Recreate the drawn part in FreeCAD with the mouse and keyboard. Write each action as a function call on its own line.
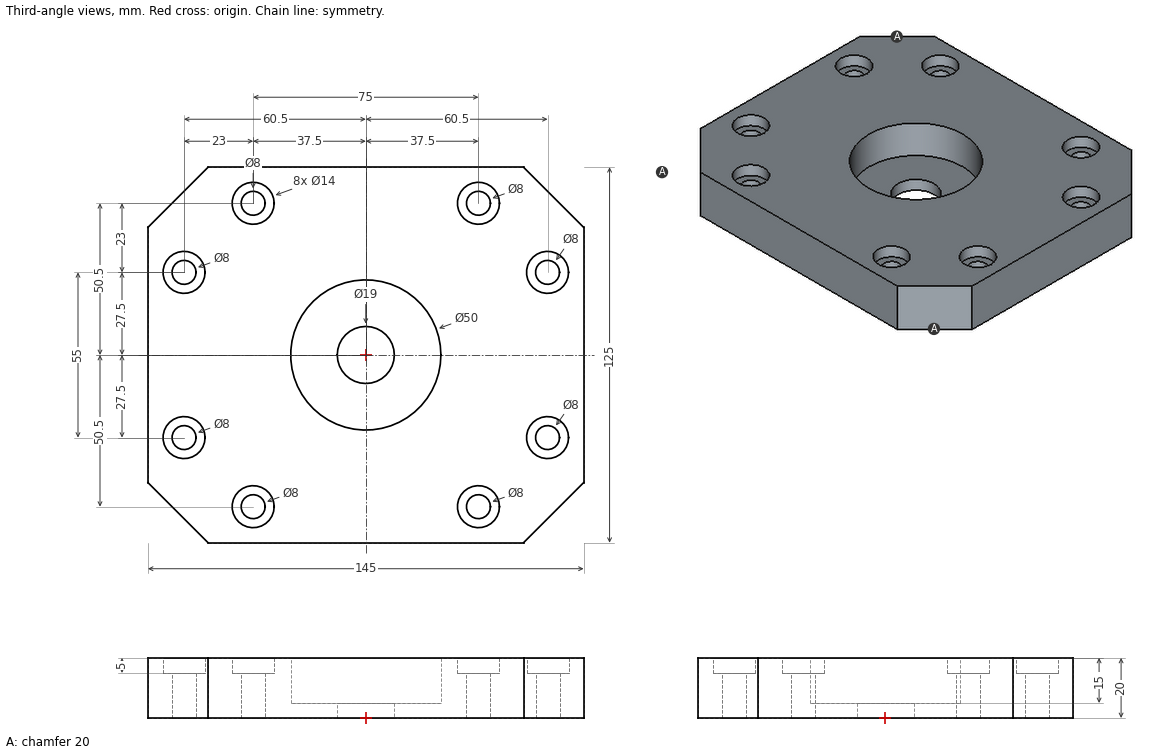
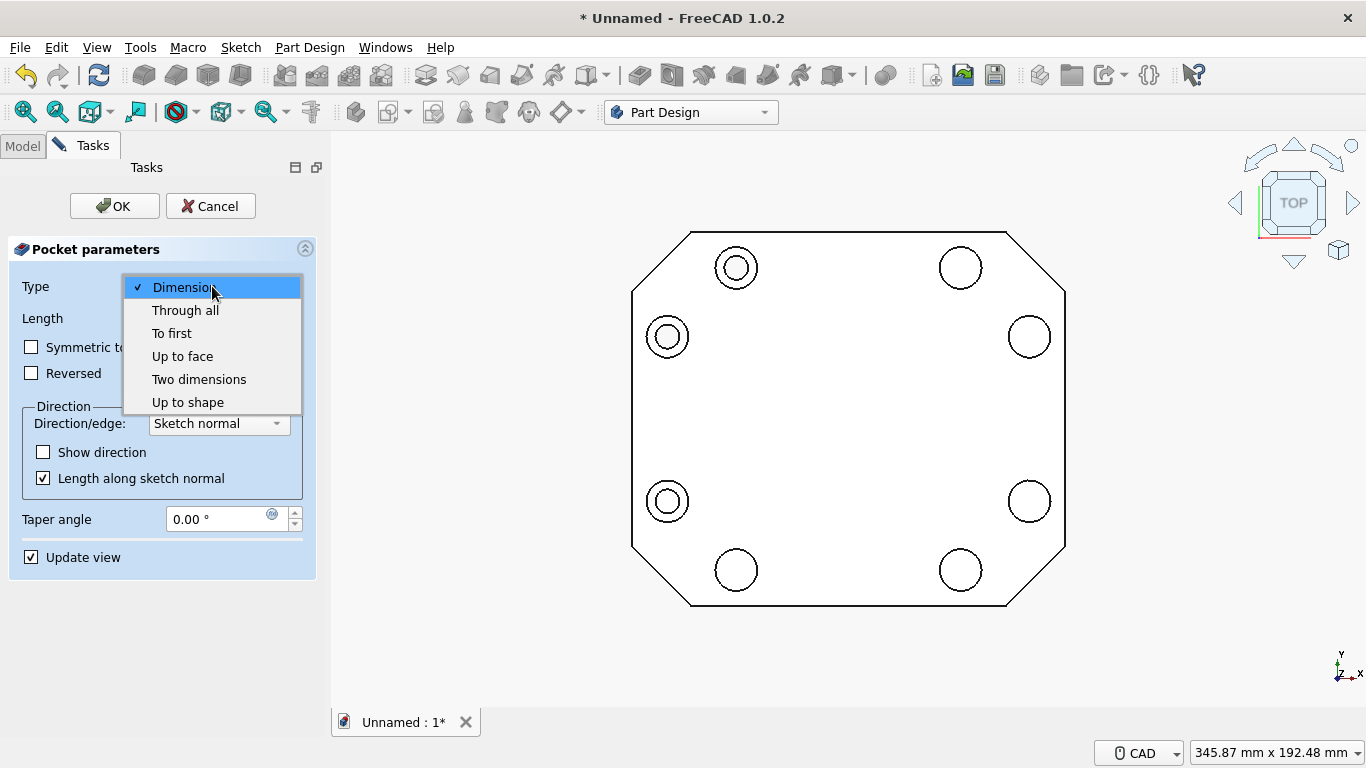
click(212, 334)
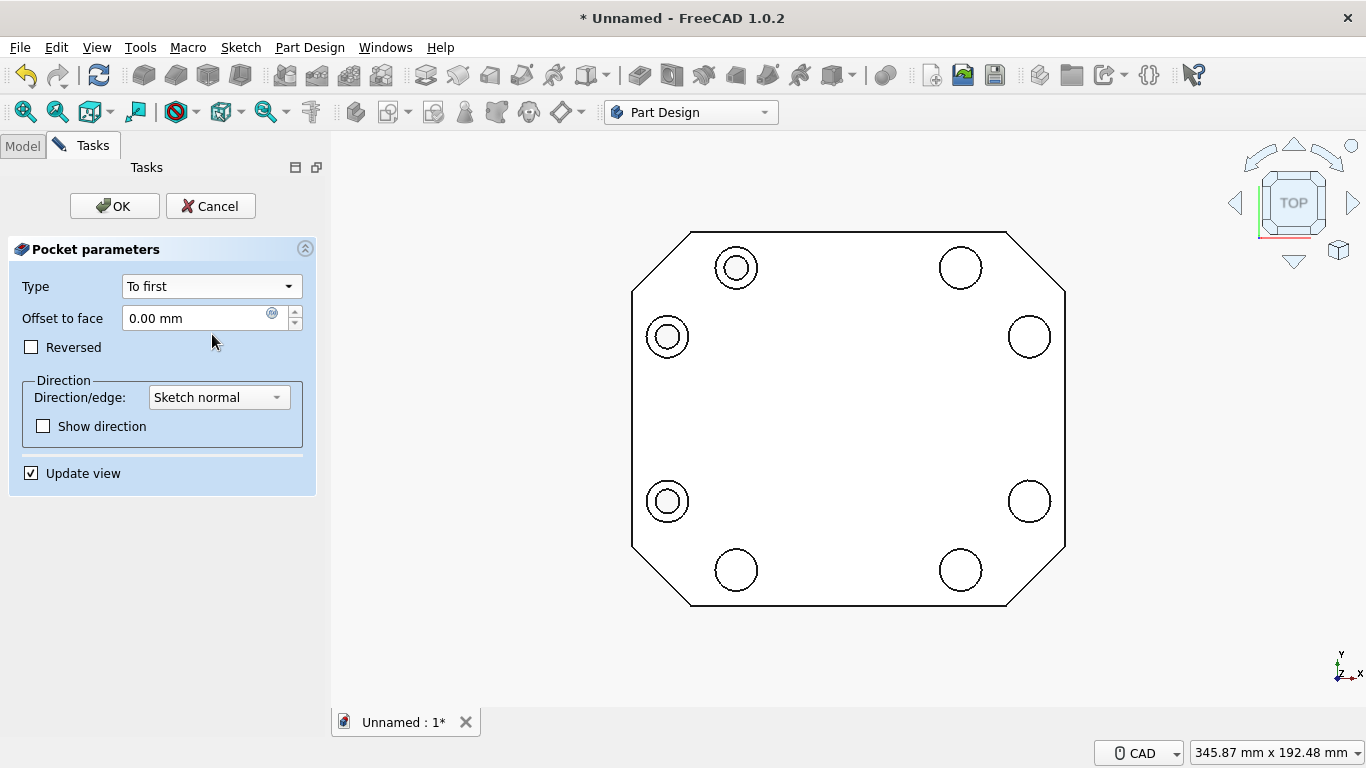
click(115, 206)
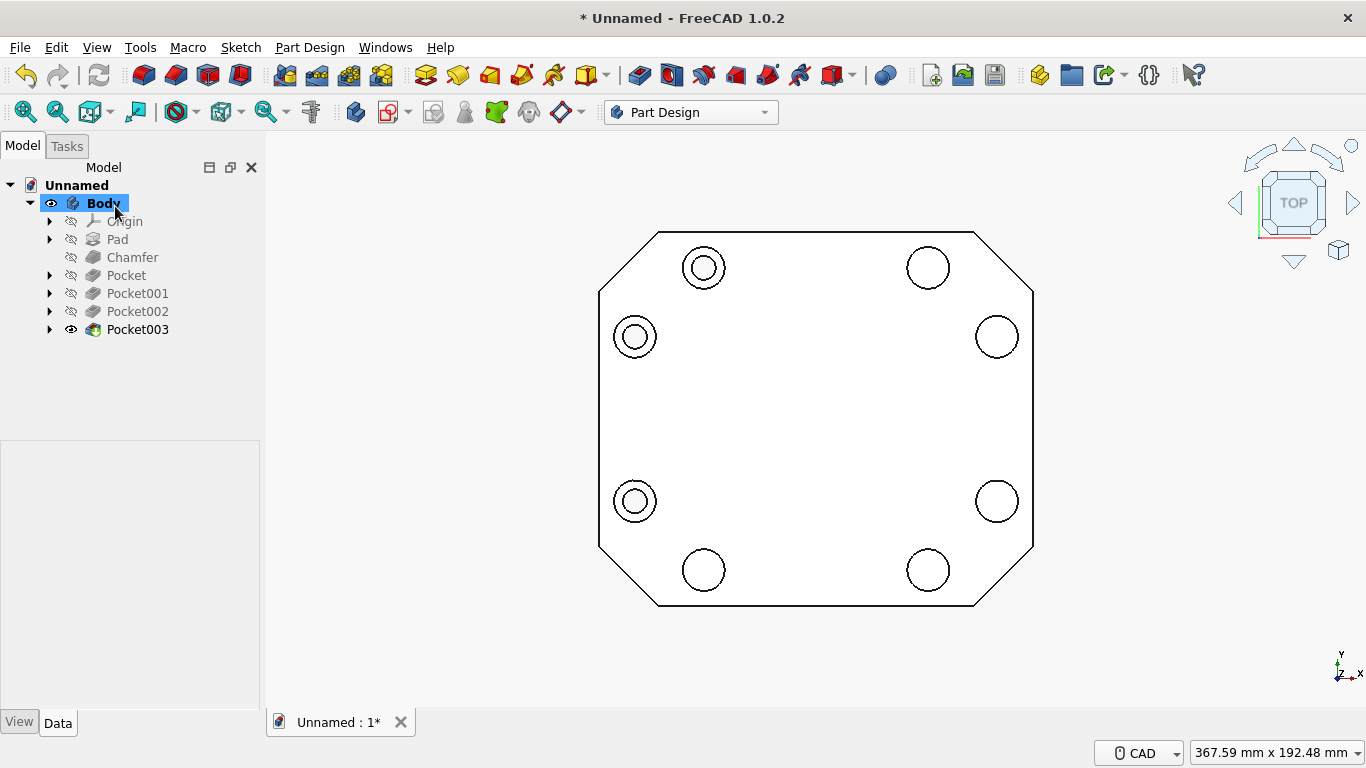
click(928, 267)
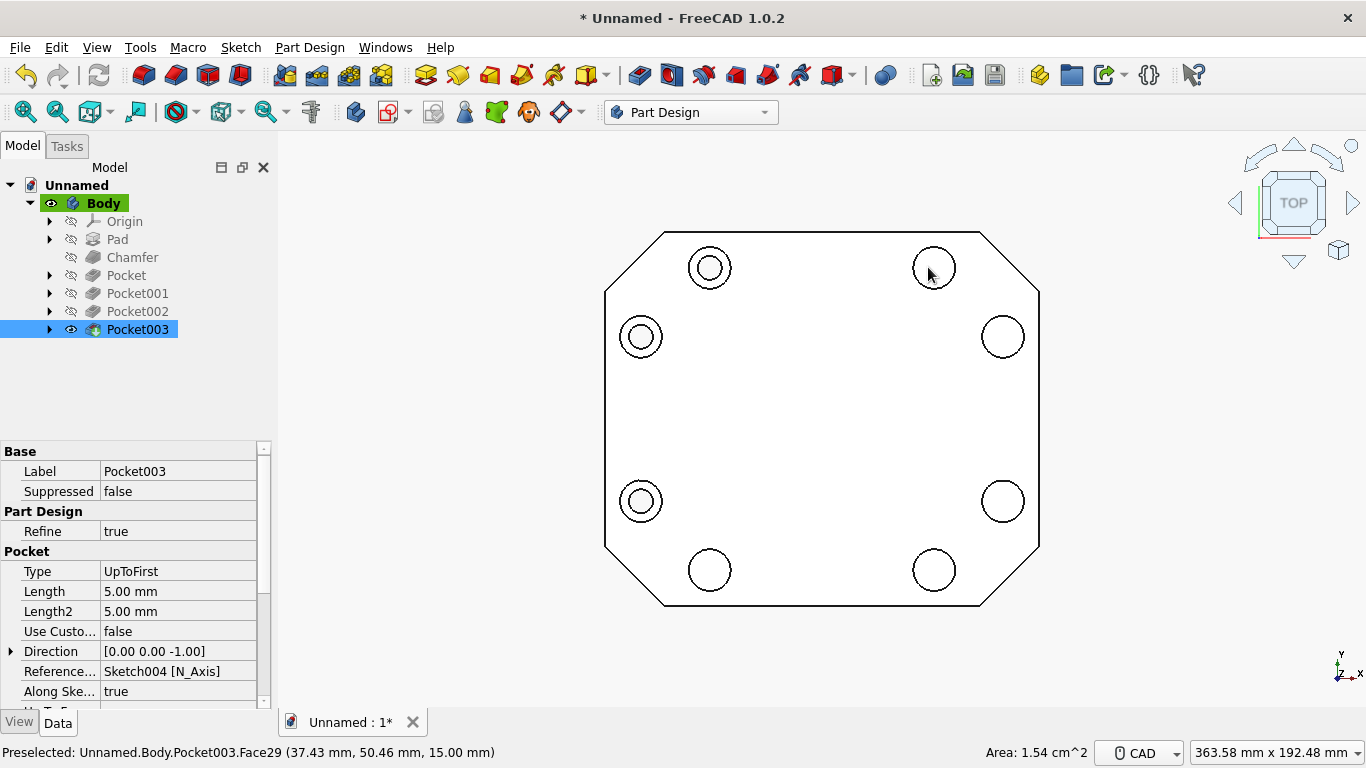
click(388, 112)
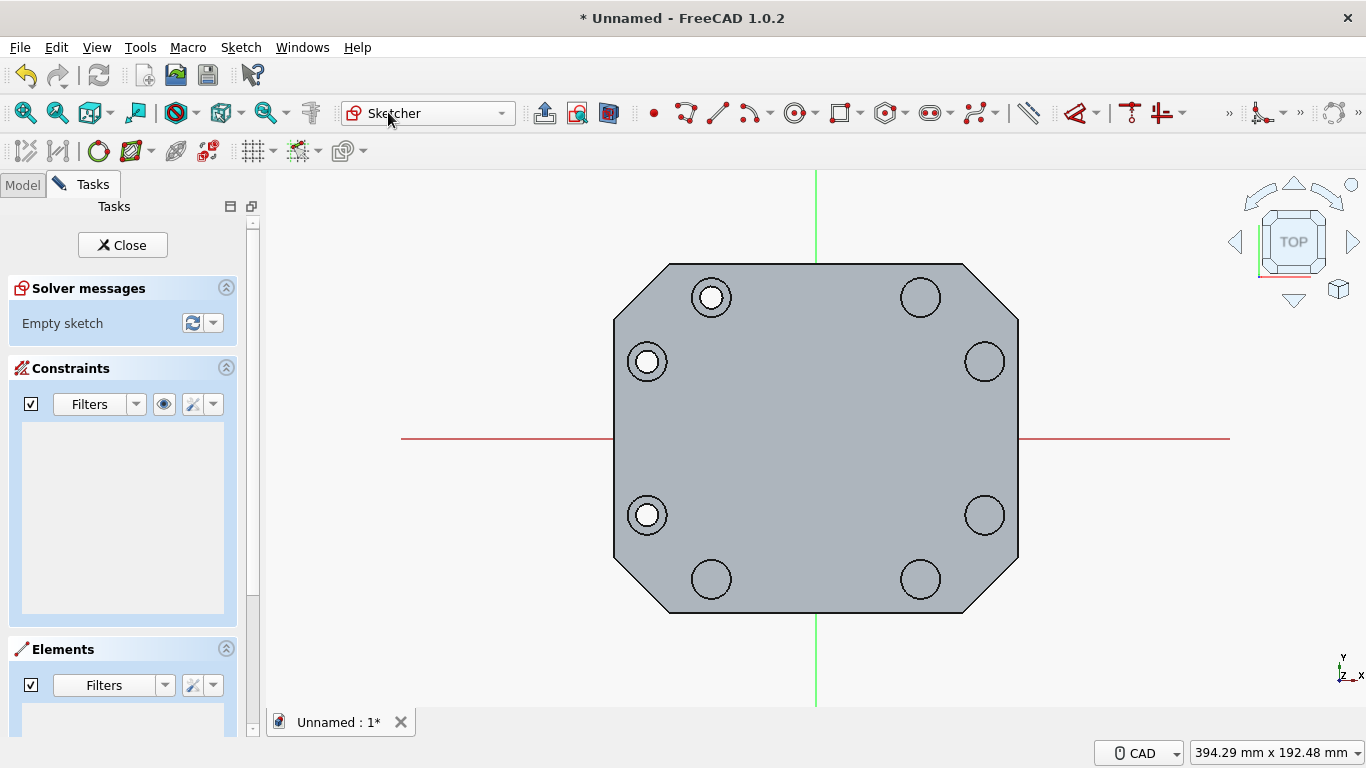
scroll(709, 589, up, 14)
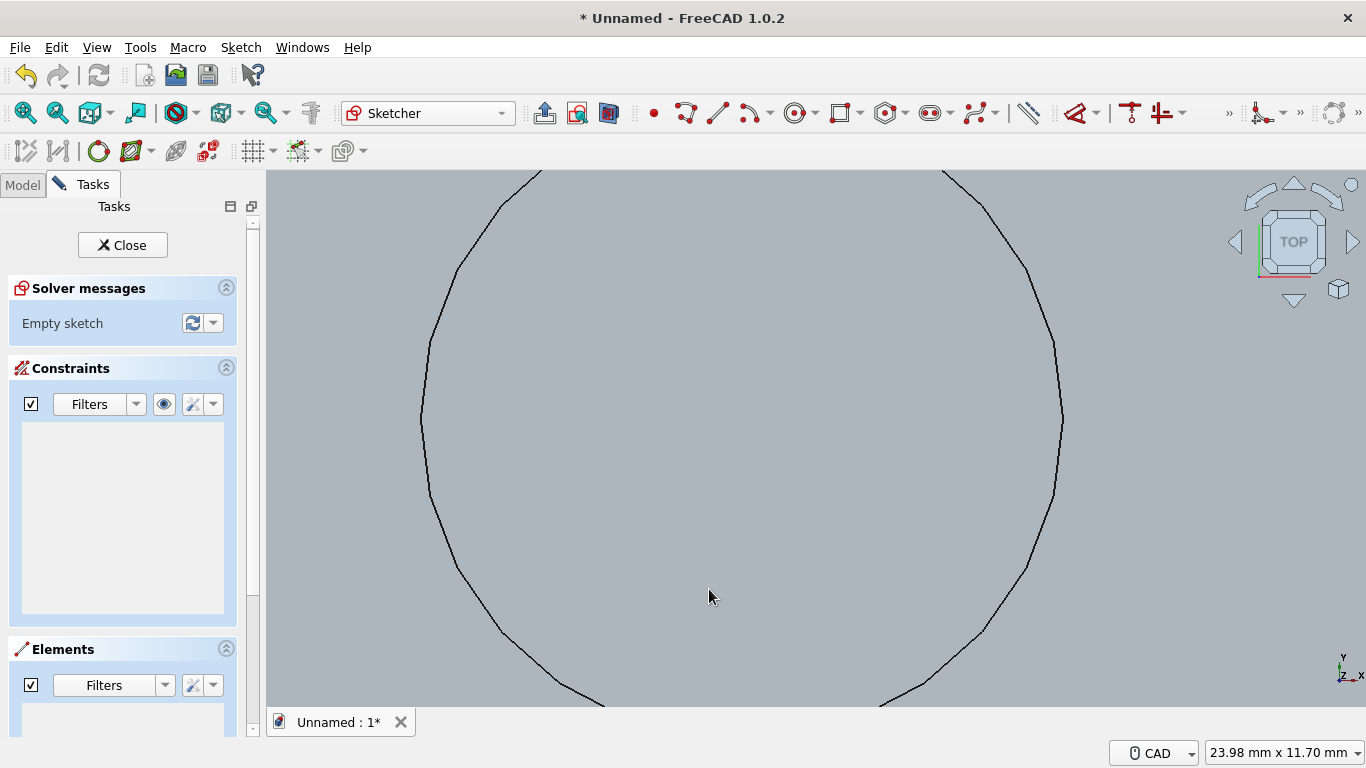
click(796, 114)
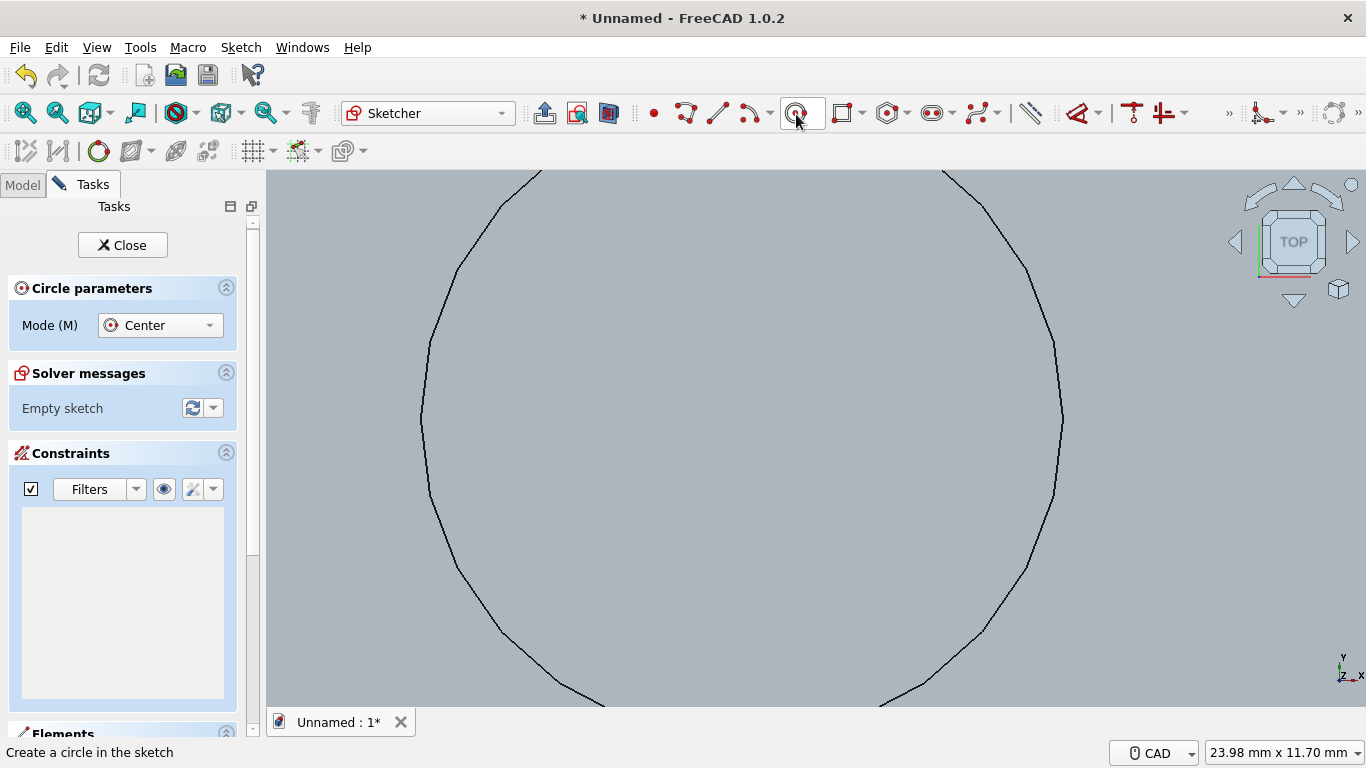
click(742, 419)
click(872, 289)
key(Escape)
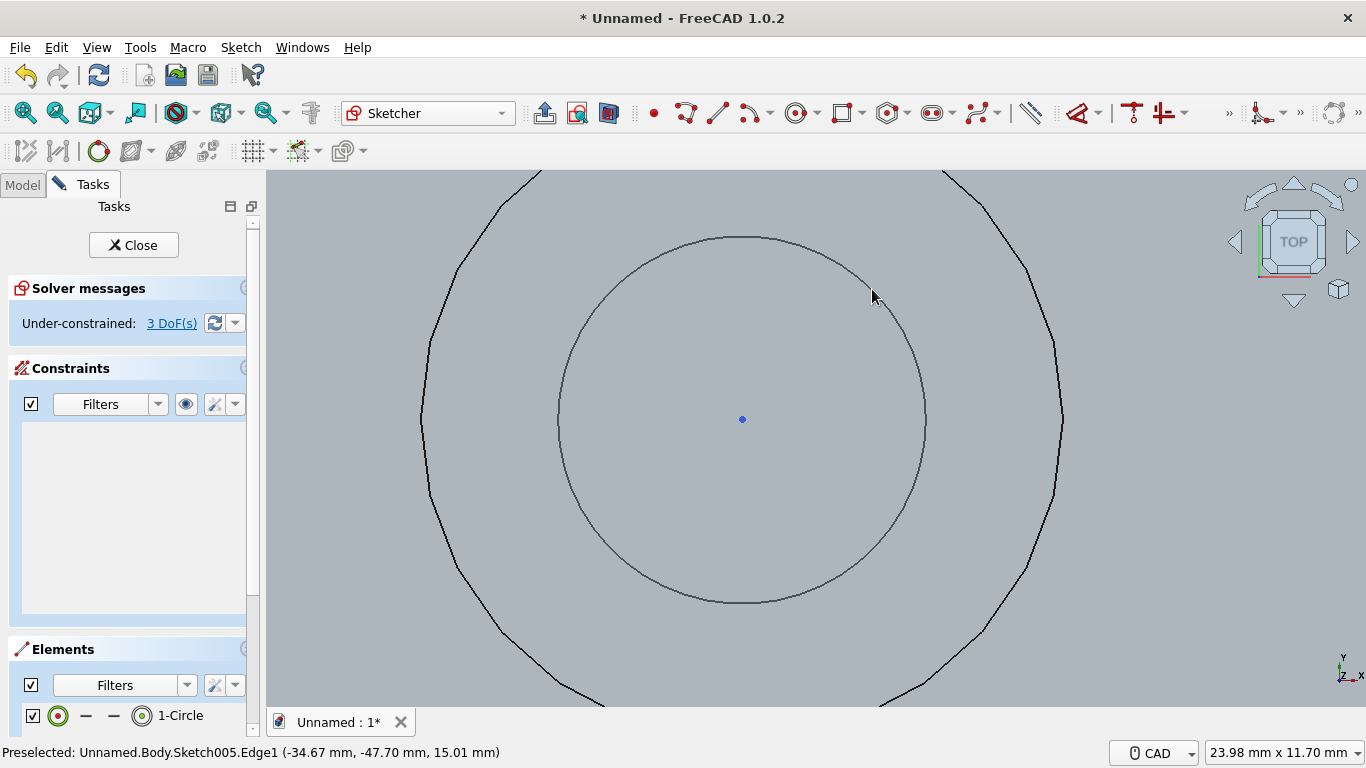
click(1078, 114)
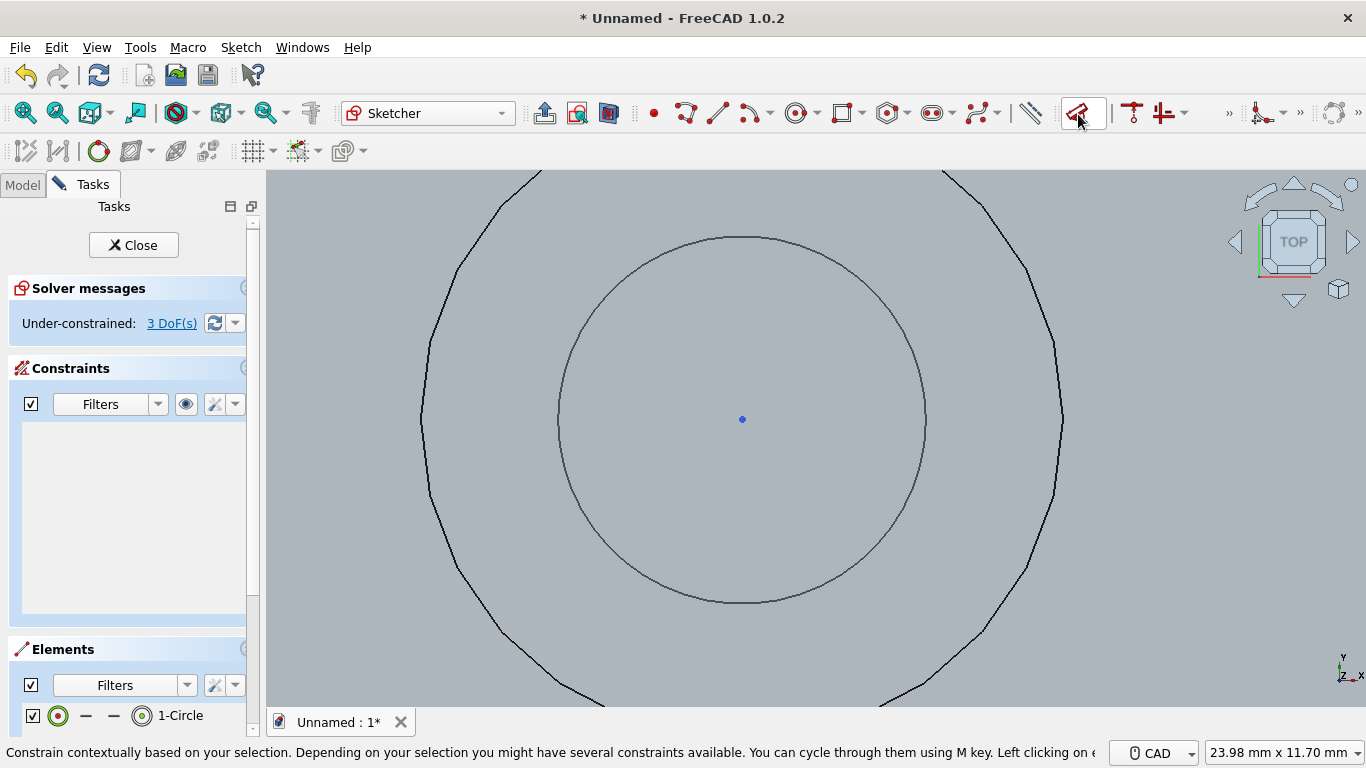
click(872, 290)
click(895, 267)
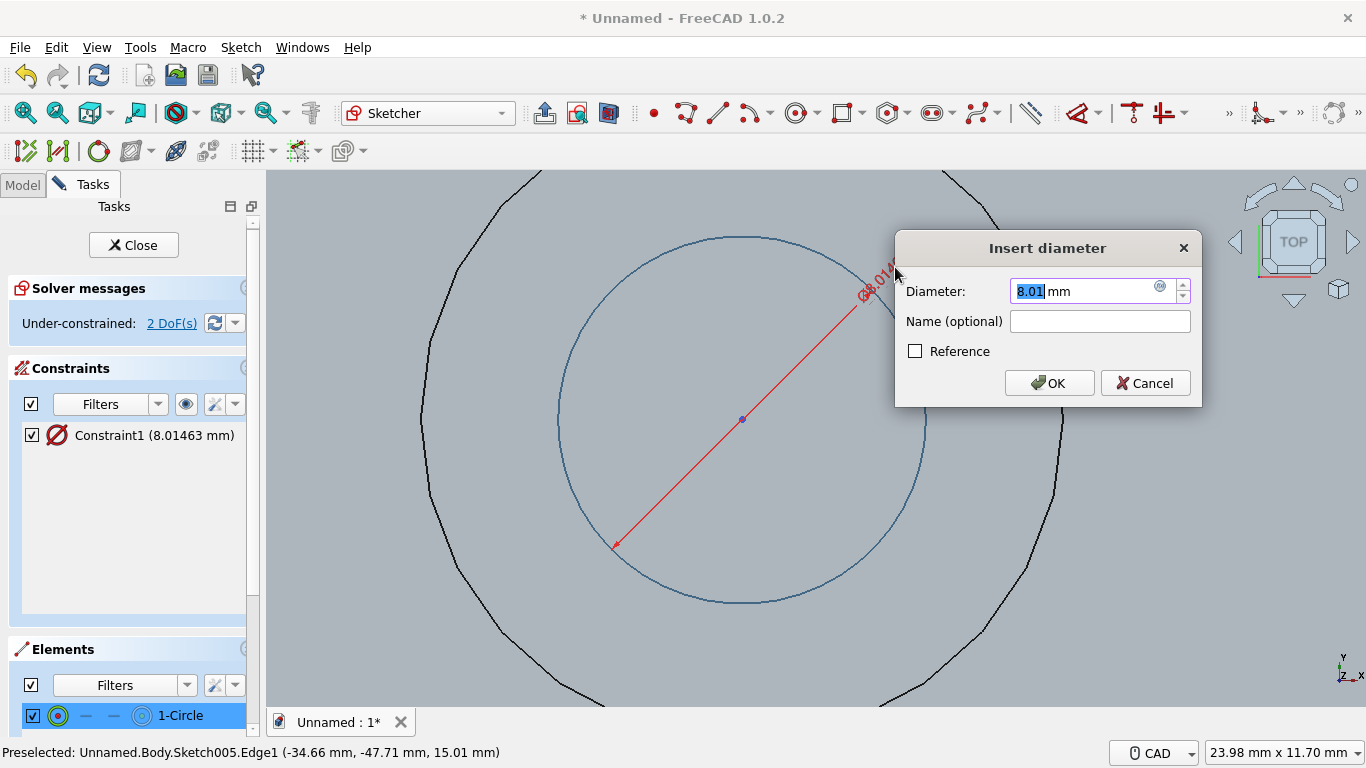
text(8)
key(Return)